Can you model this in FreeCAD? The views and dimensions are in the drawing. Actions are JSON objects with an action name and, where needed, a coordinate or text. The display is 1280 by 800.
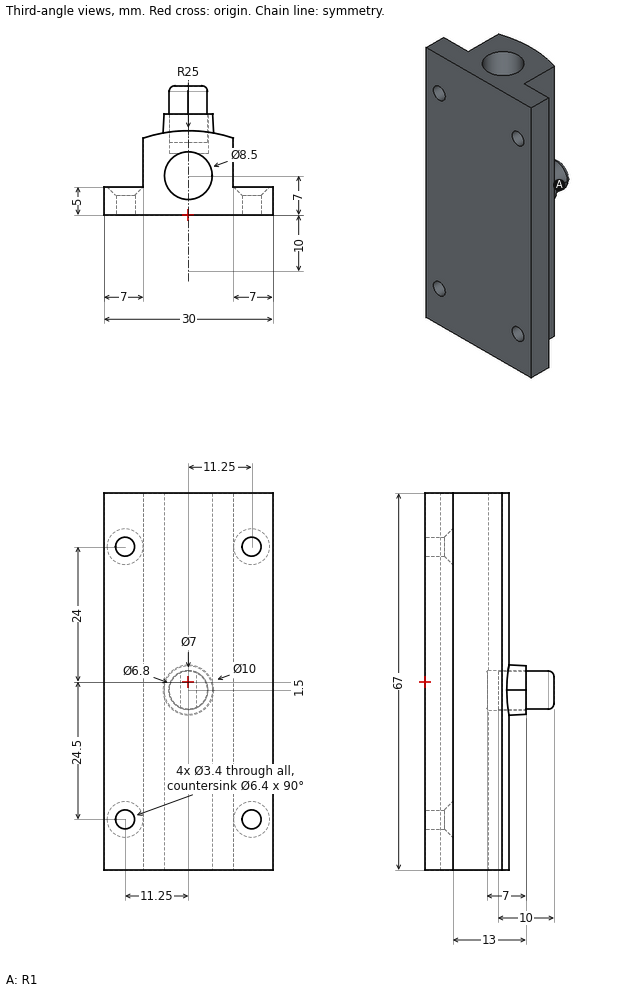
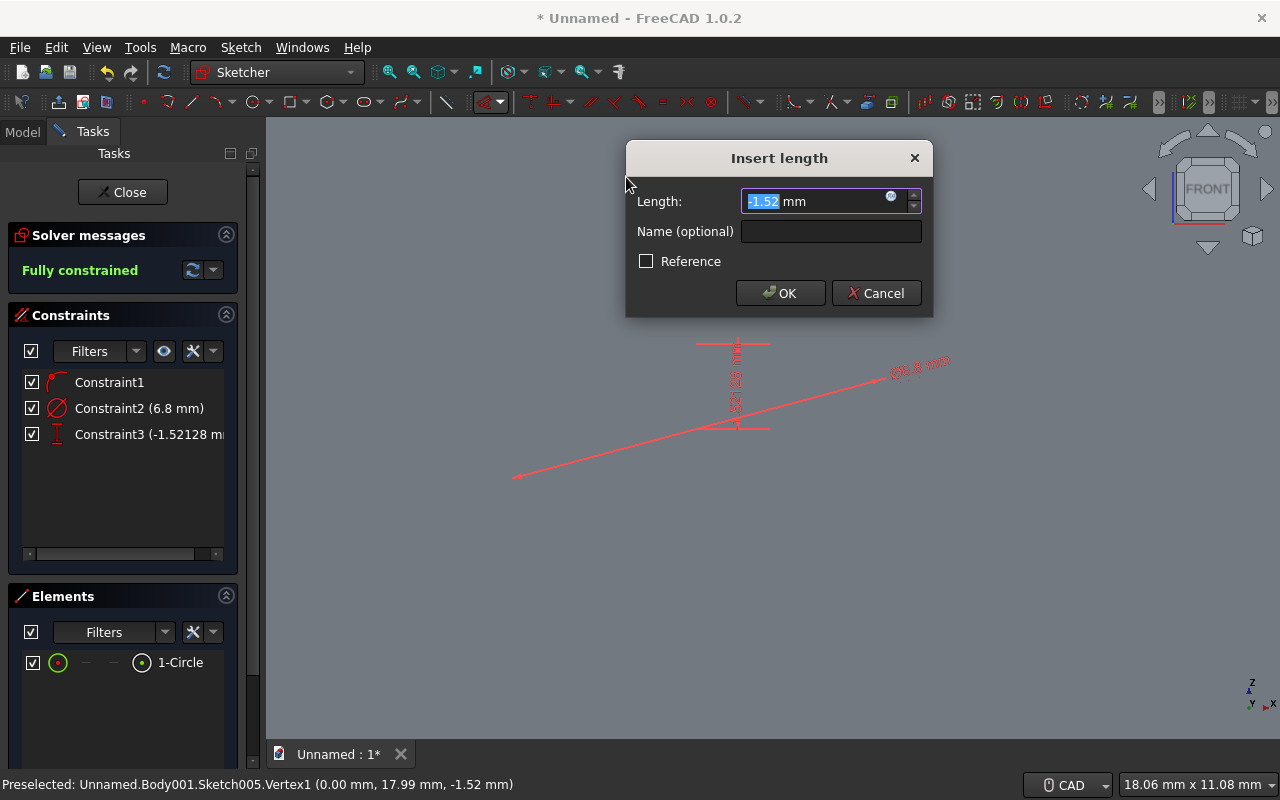
{"action": "type", "text": "-1.5"}
{"action": "key", "text": "Return"}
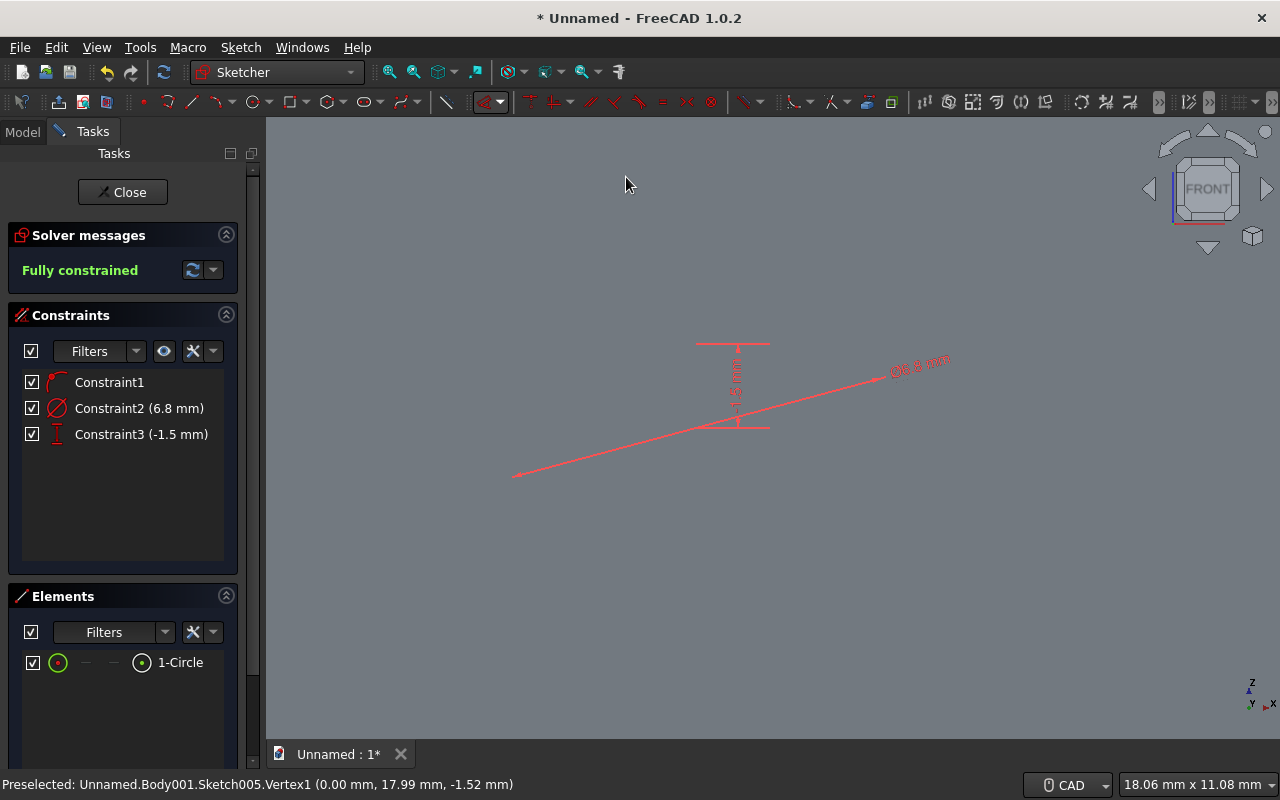
{"action": "left_click", "coordinate": [123, 192]}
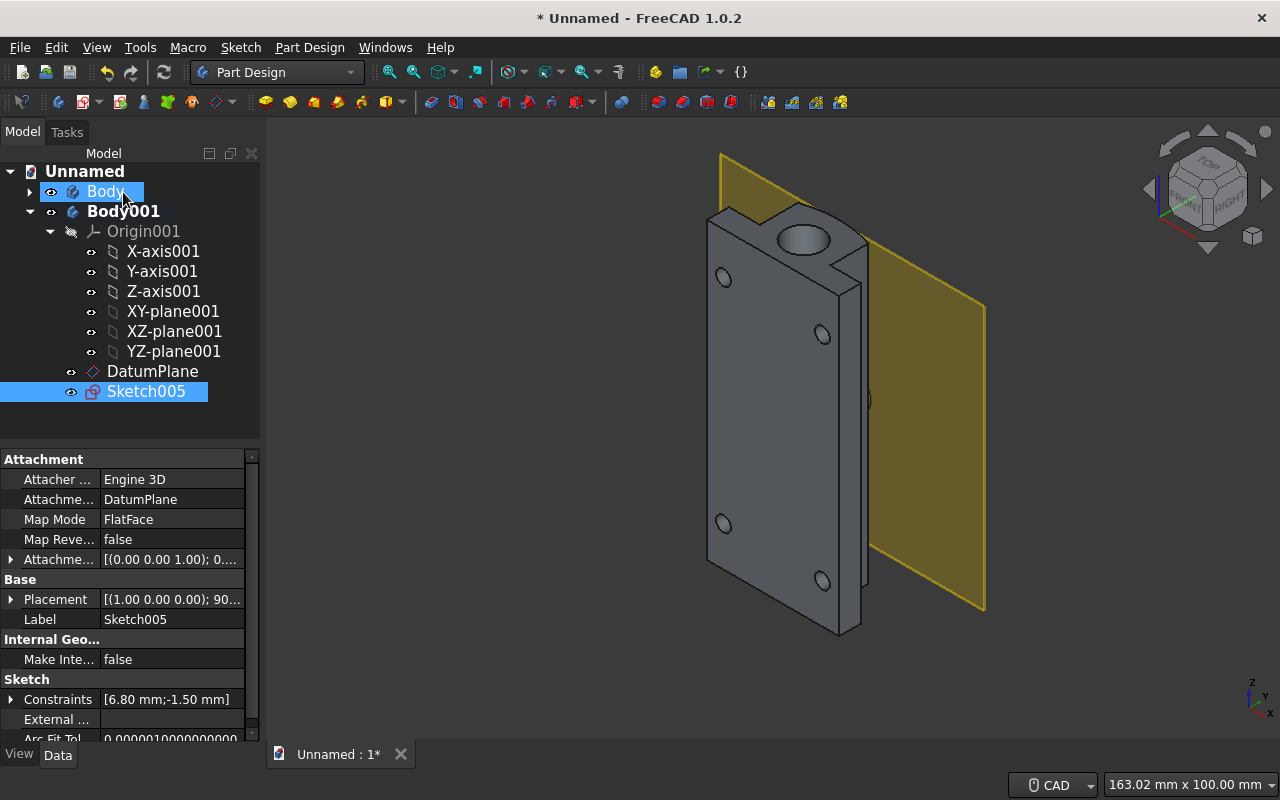
{"action": "left_click", "coordinate": [266, 102]}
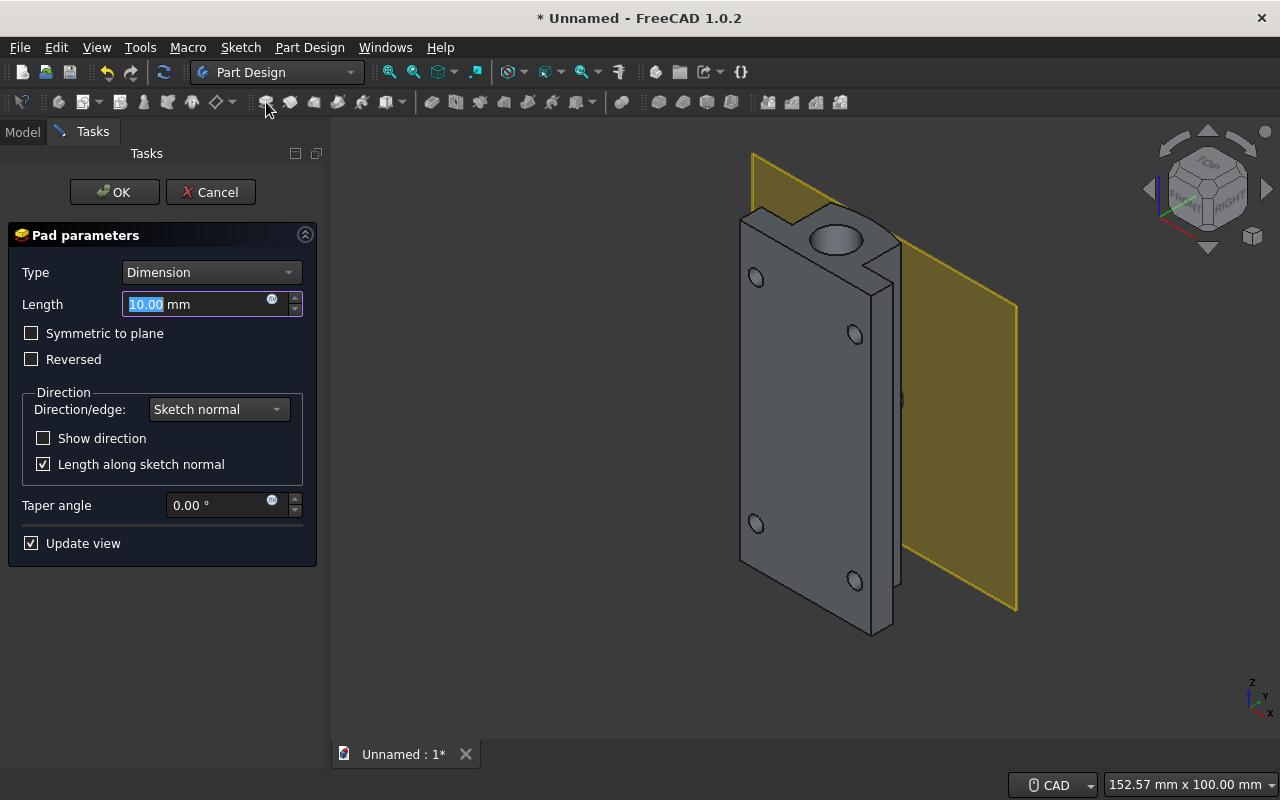
{"action": "type", "text": "10"}
{"action": "key", "text": "Tab"}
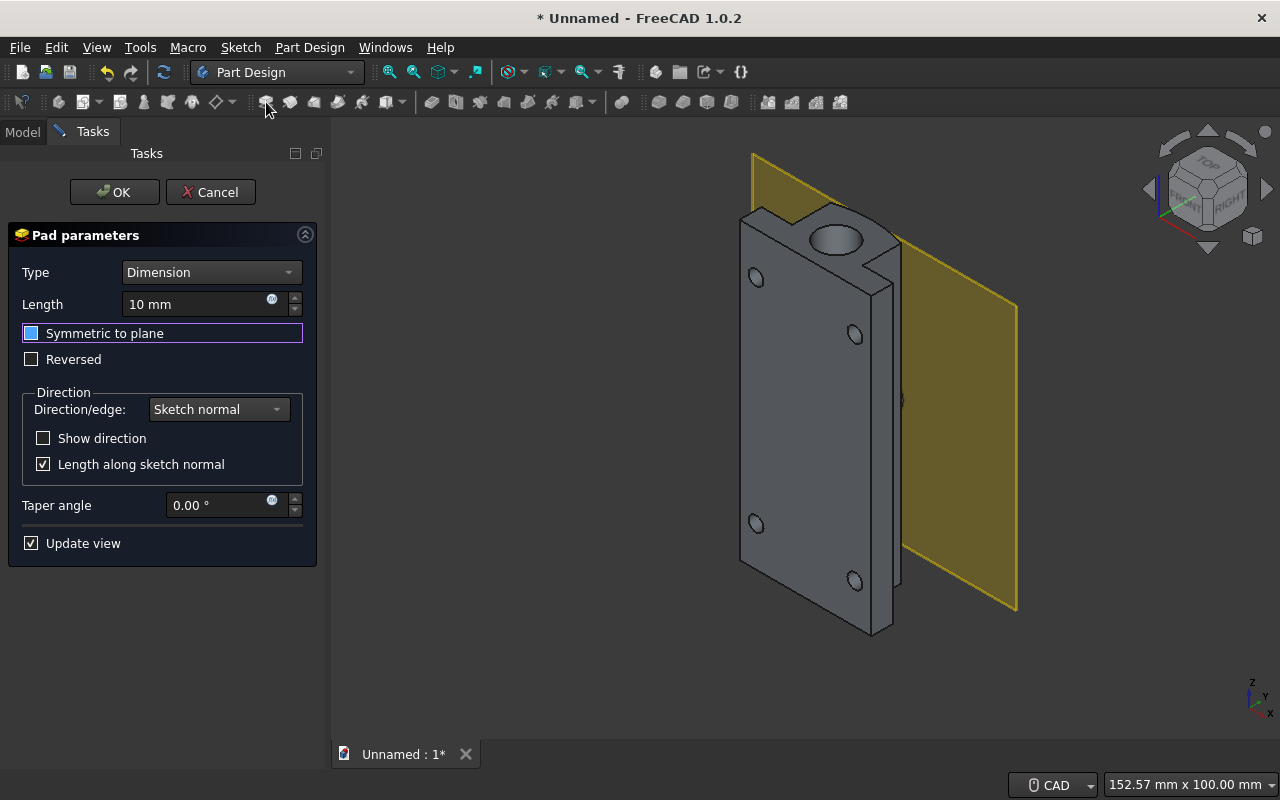
{"action": "left_click", "coordinate": [30, 333]}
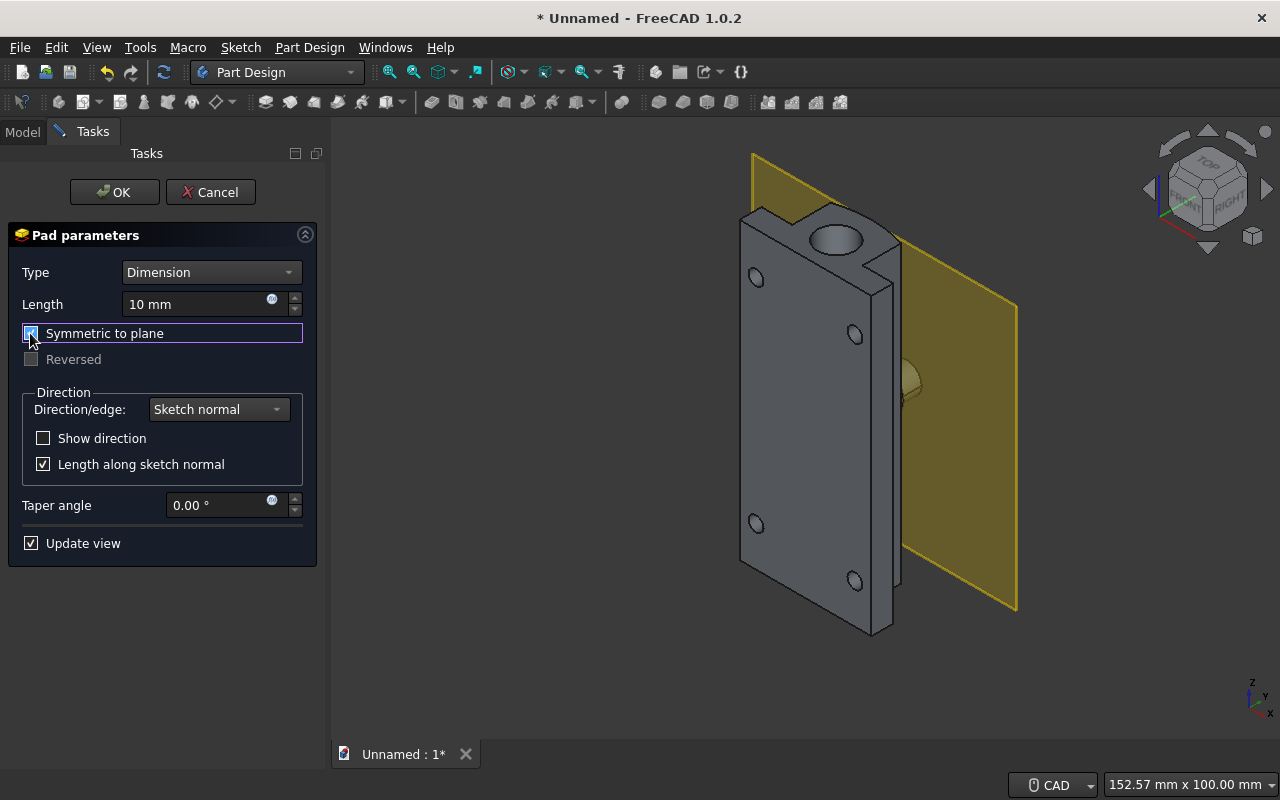
{"action": "left_click", "coordinate": [115, 192]}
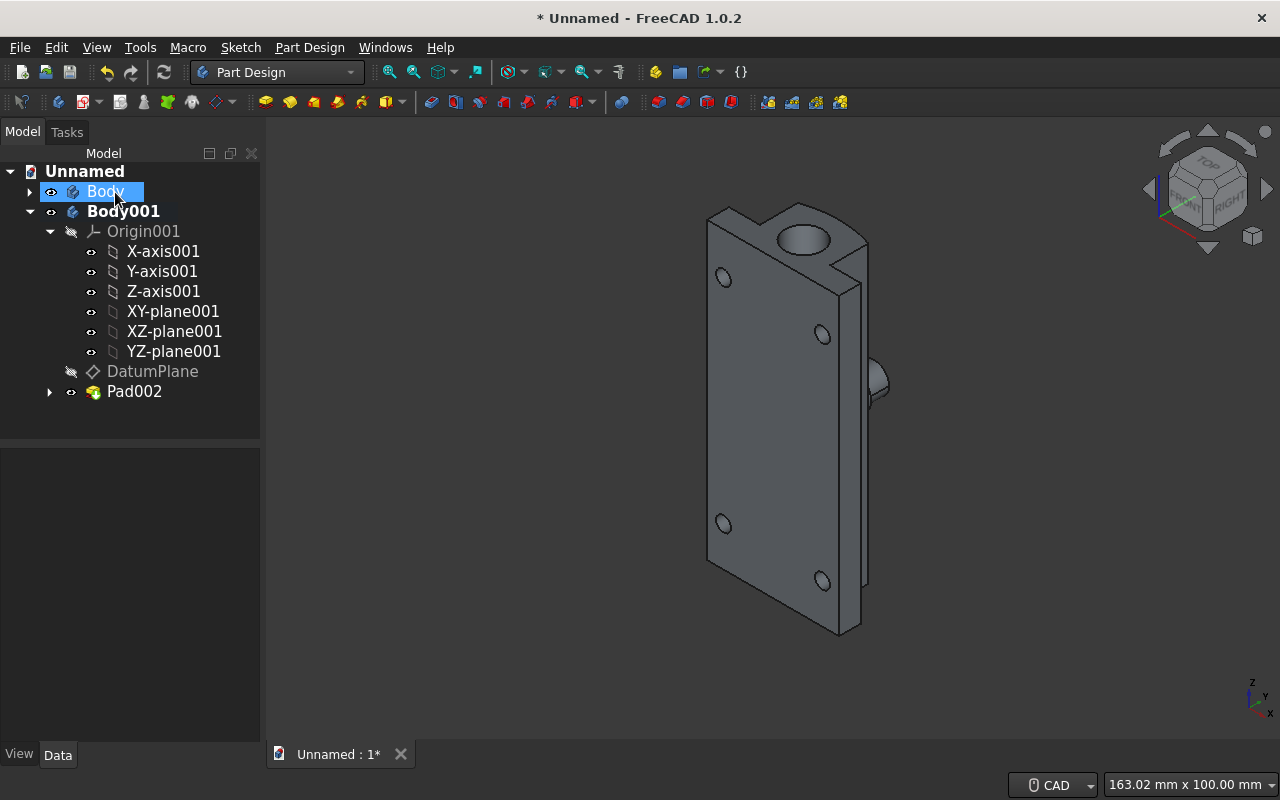
{"action": "left_click", "coordinate": [390, 72]}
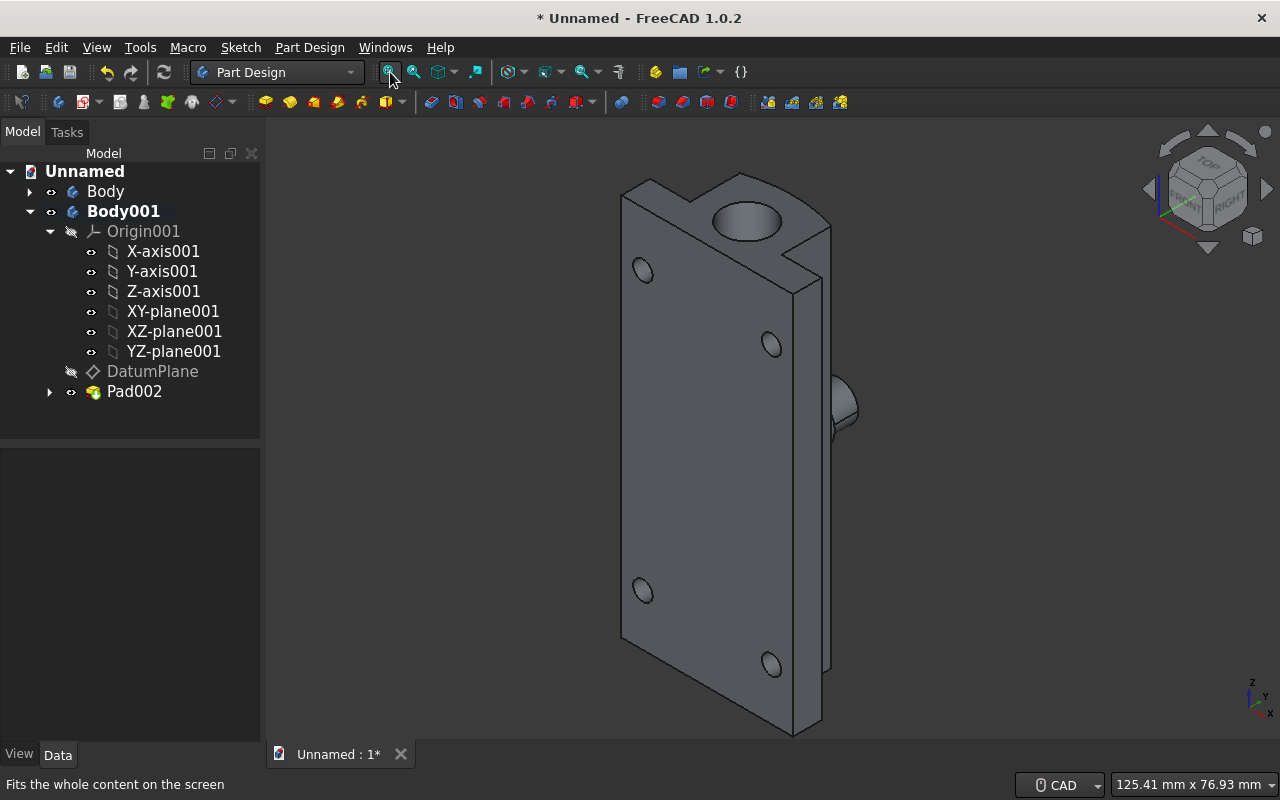
{"action": "left_click", "coordinate": [845, 381]}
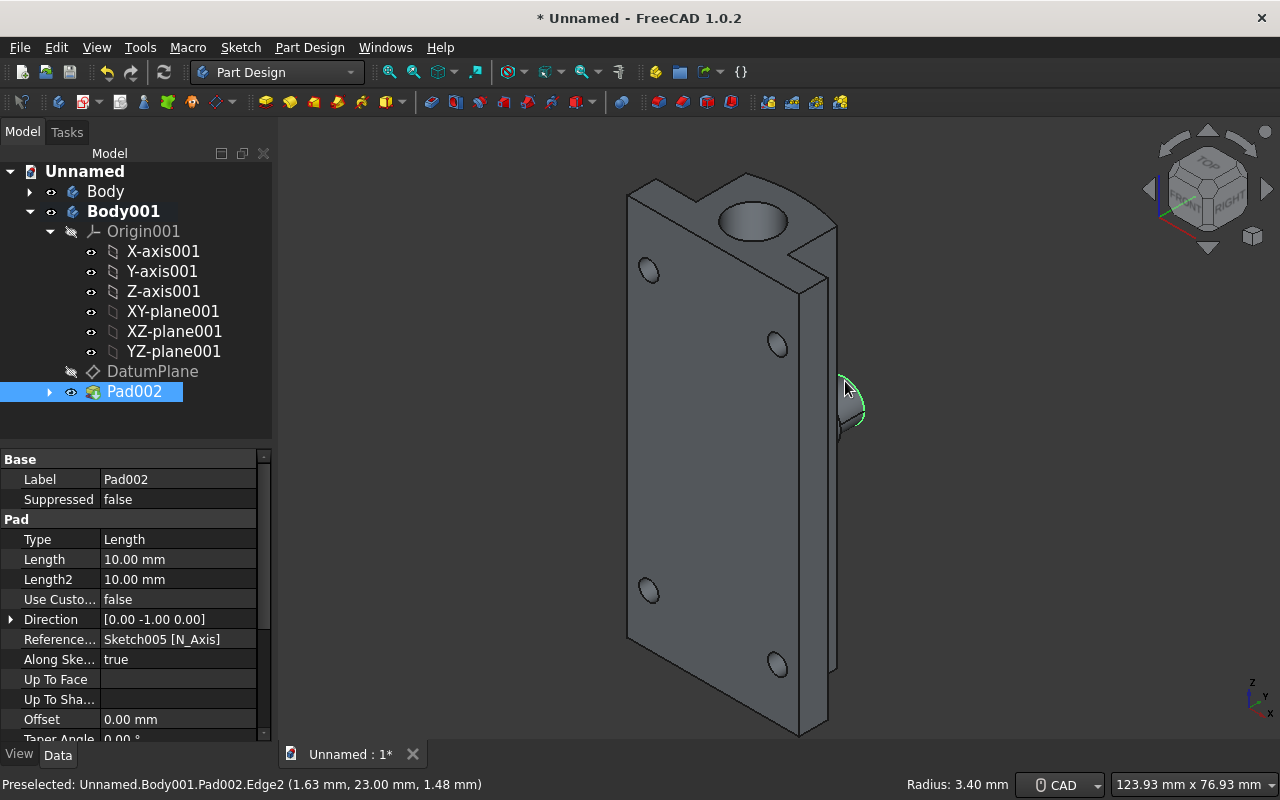
{"action": "left_click", "coordinate": [660, 102]}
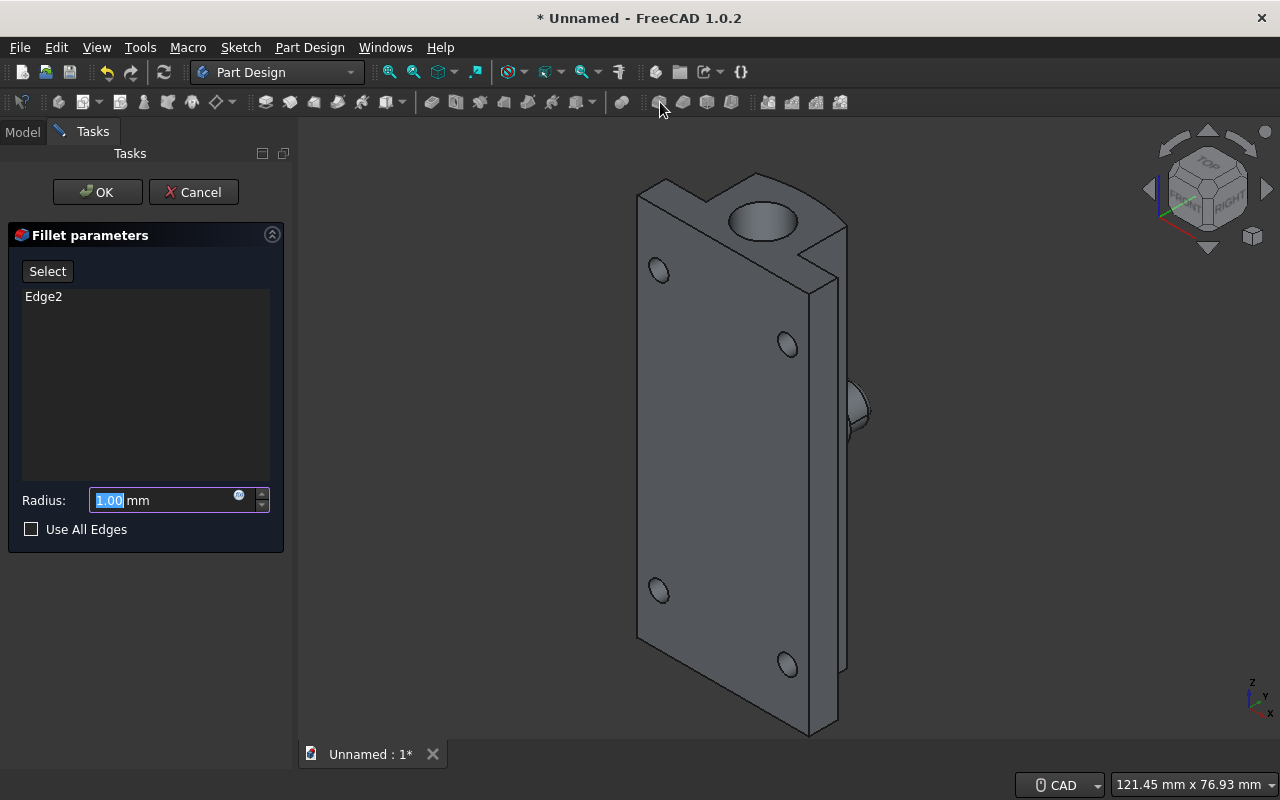
{"action": "type", "text": "1"}
{"action": "key", "text": "Tab"}